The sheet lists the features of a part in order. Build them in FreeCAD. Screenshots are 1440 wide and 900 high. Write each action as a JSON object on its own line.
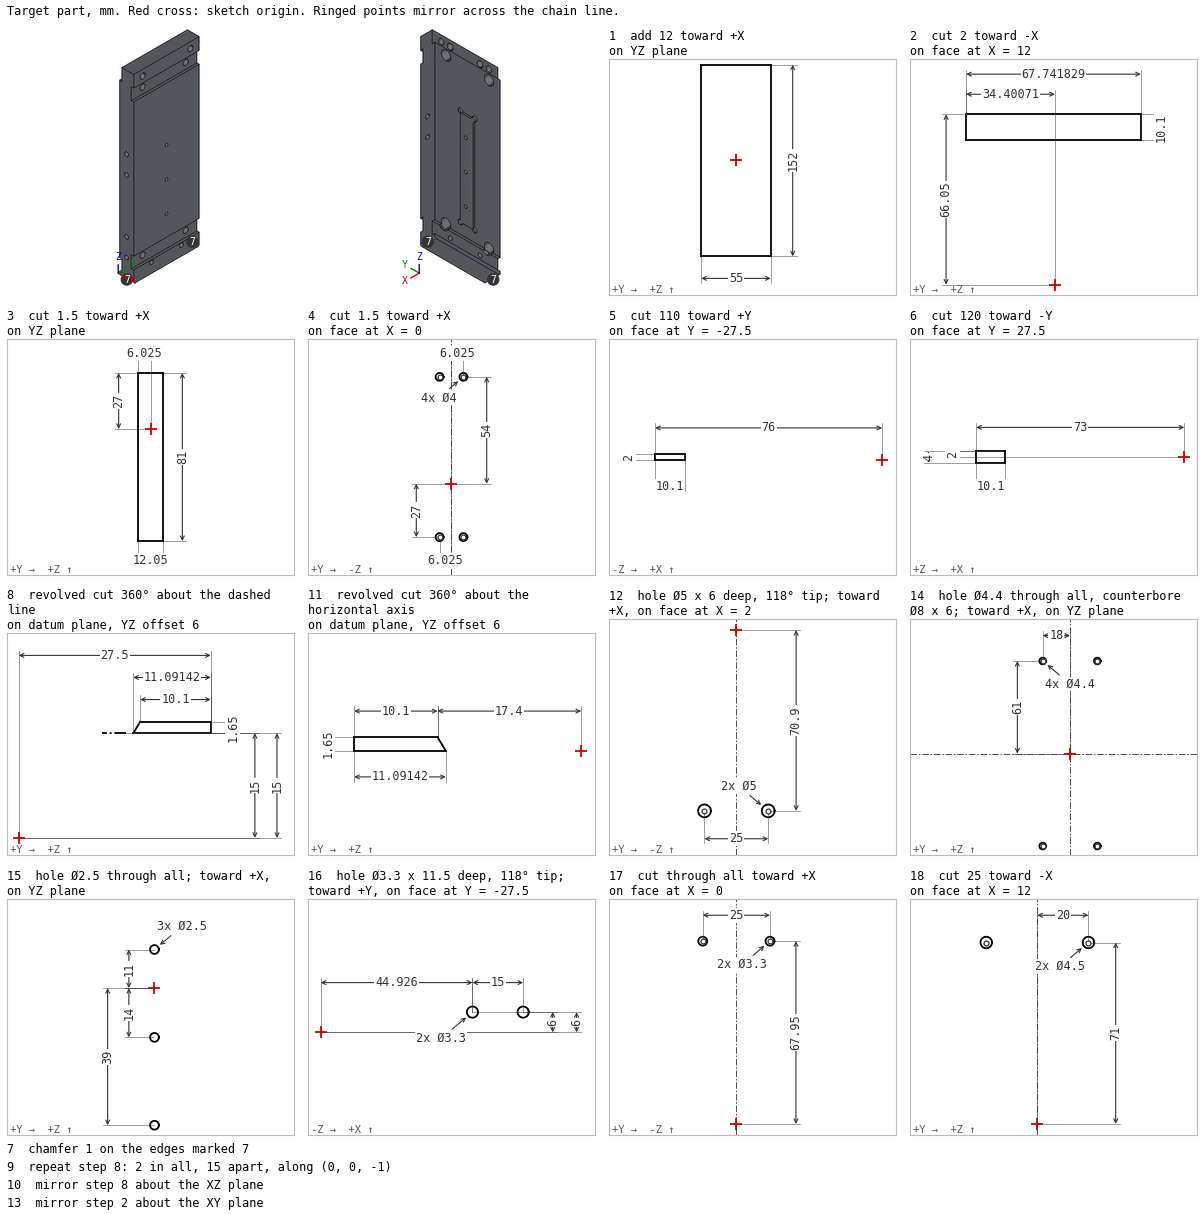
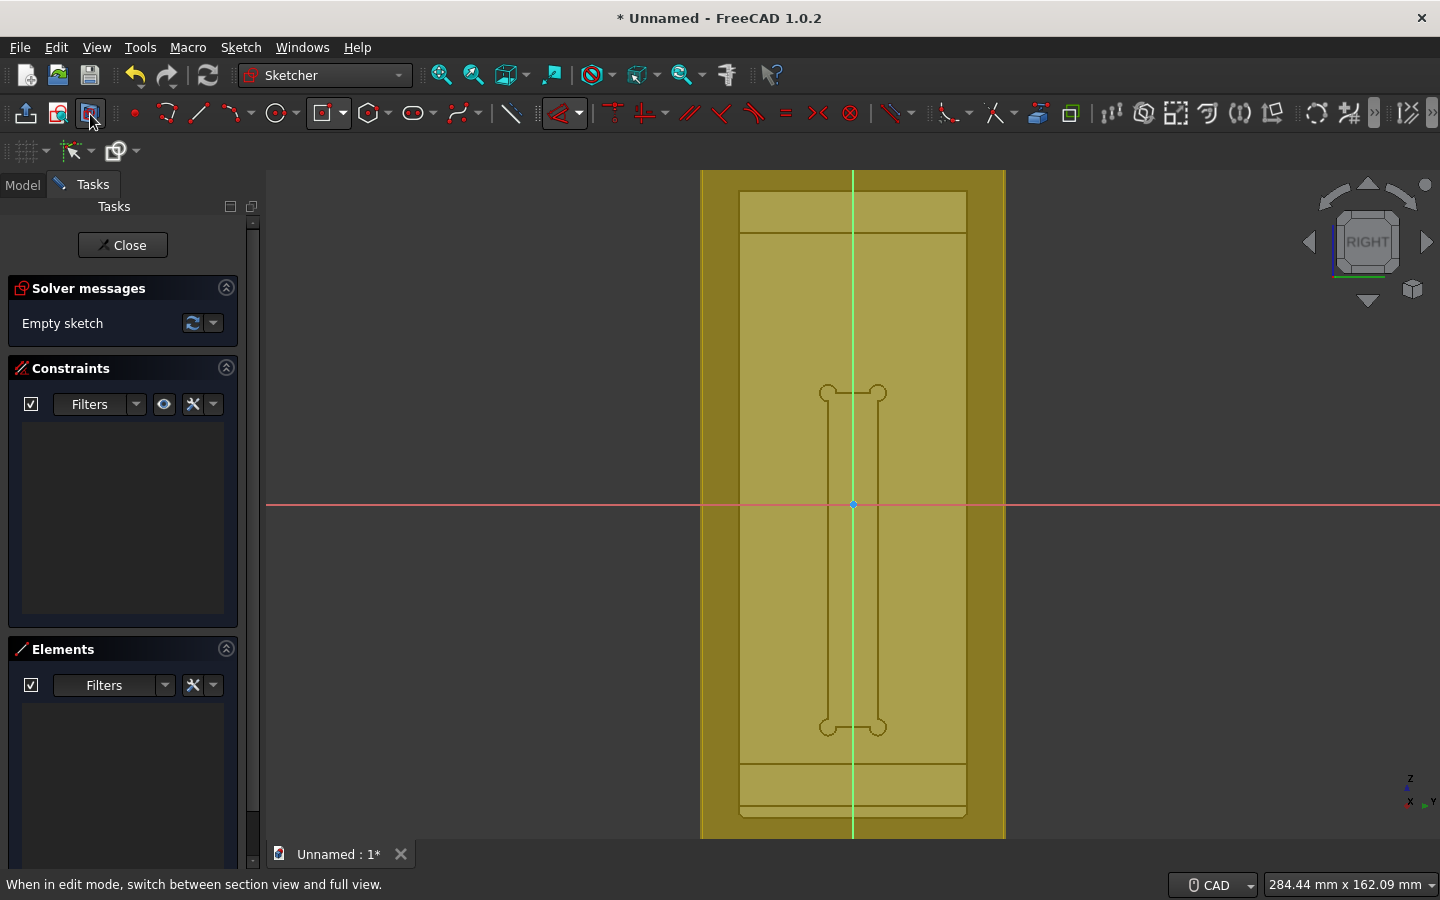
{"action": "scroll", "coordinate": [935, 463], "scroll_direction": "up", "scroll_amount": 9}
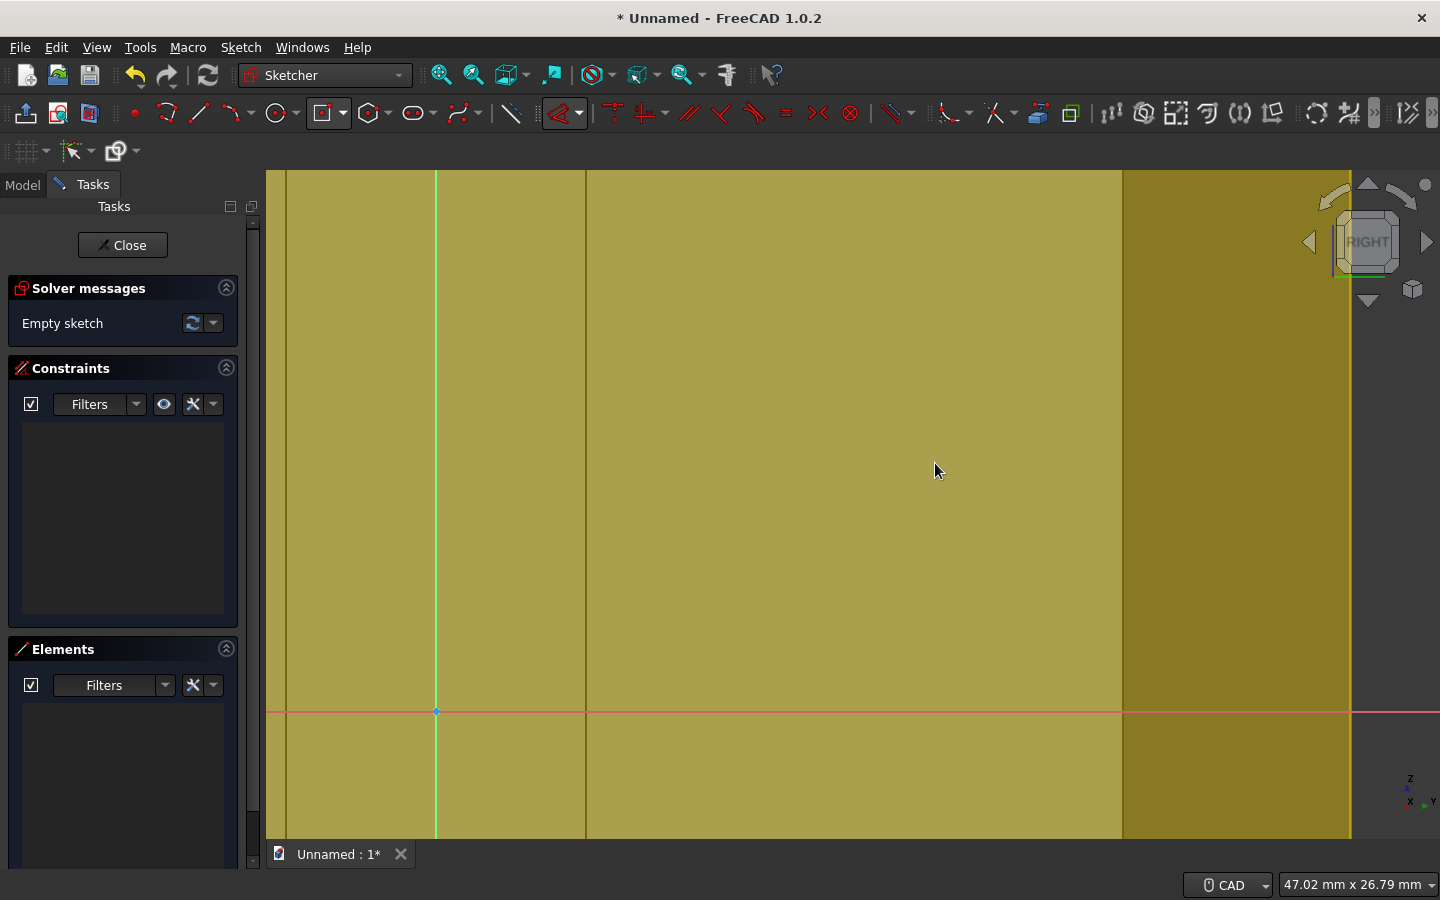
{"action": "left_click", "coordinate": [168, 114]}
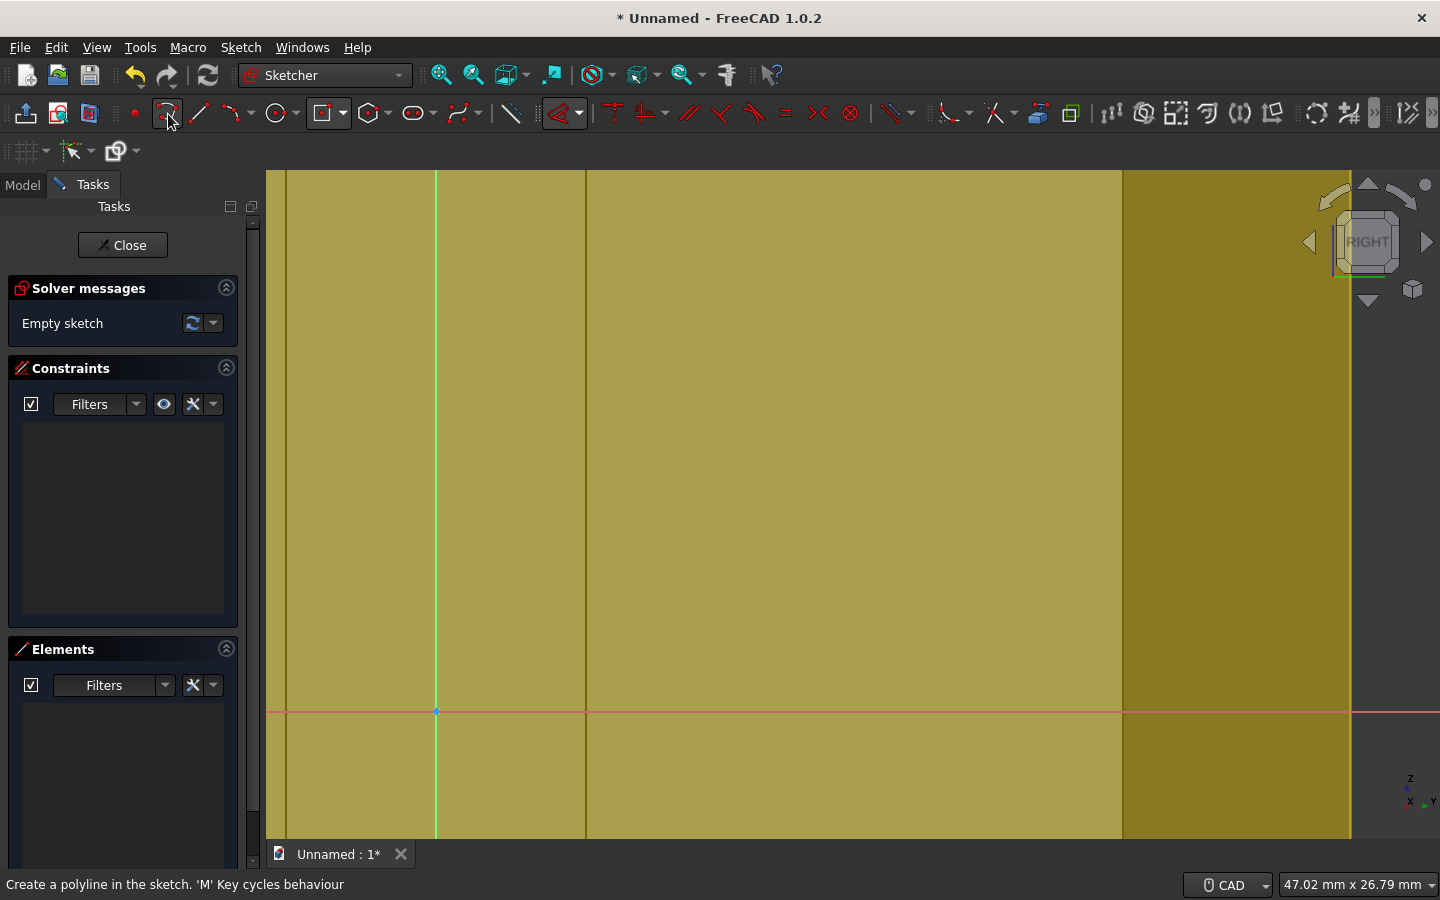
{"action": "left_click", "coordinate": [846, 337]}
{"action": "left_click", "coordinate": [1123, 337]}
{"action": "left_click", "coordinate": [1123, 296]}
{"action": "left_click", "coordinate": [871, 296]}
{"action": "left_click", "coordinate": [846, 338]}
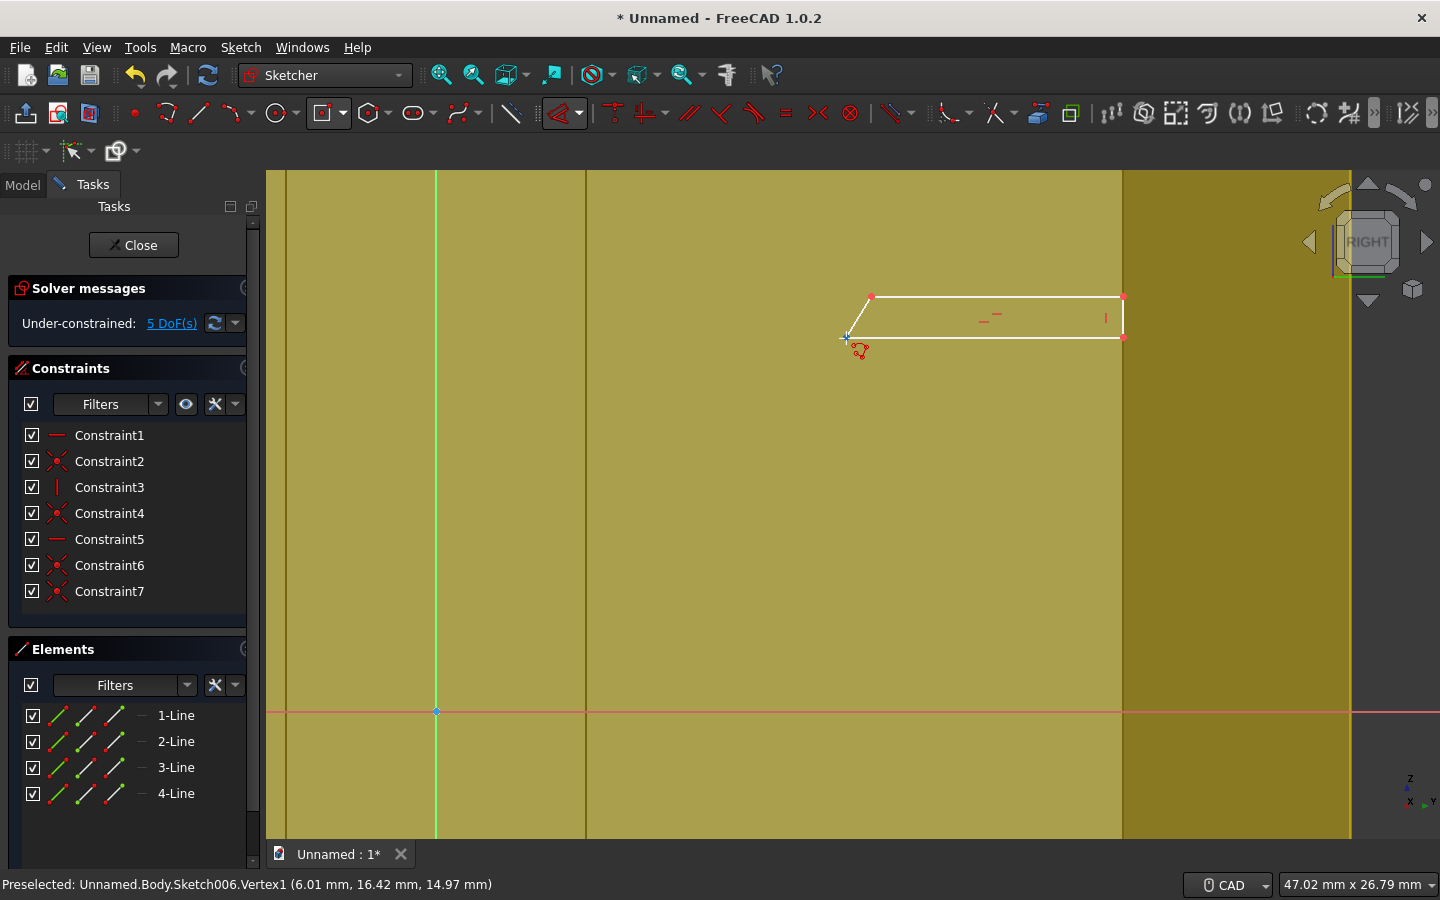
{"action": "left_click", "coordinate": [200, 114]}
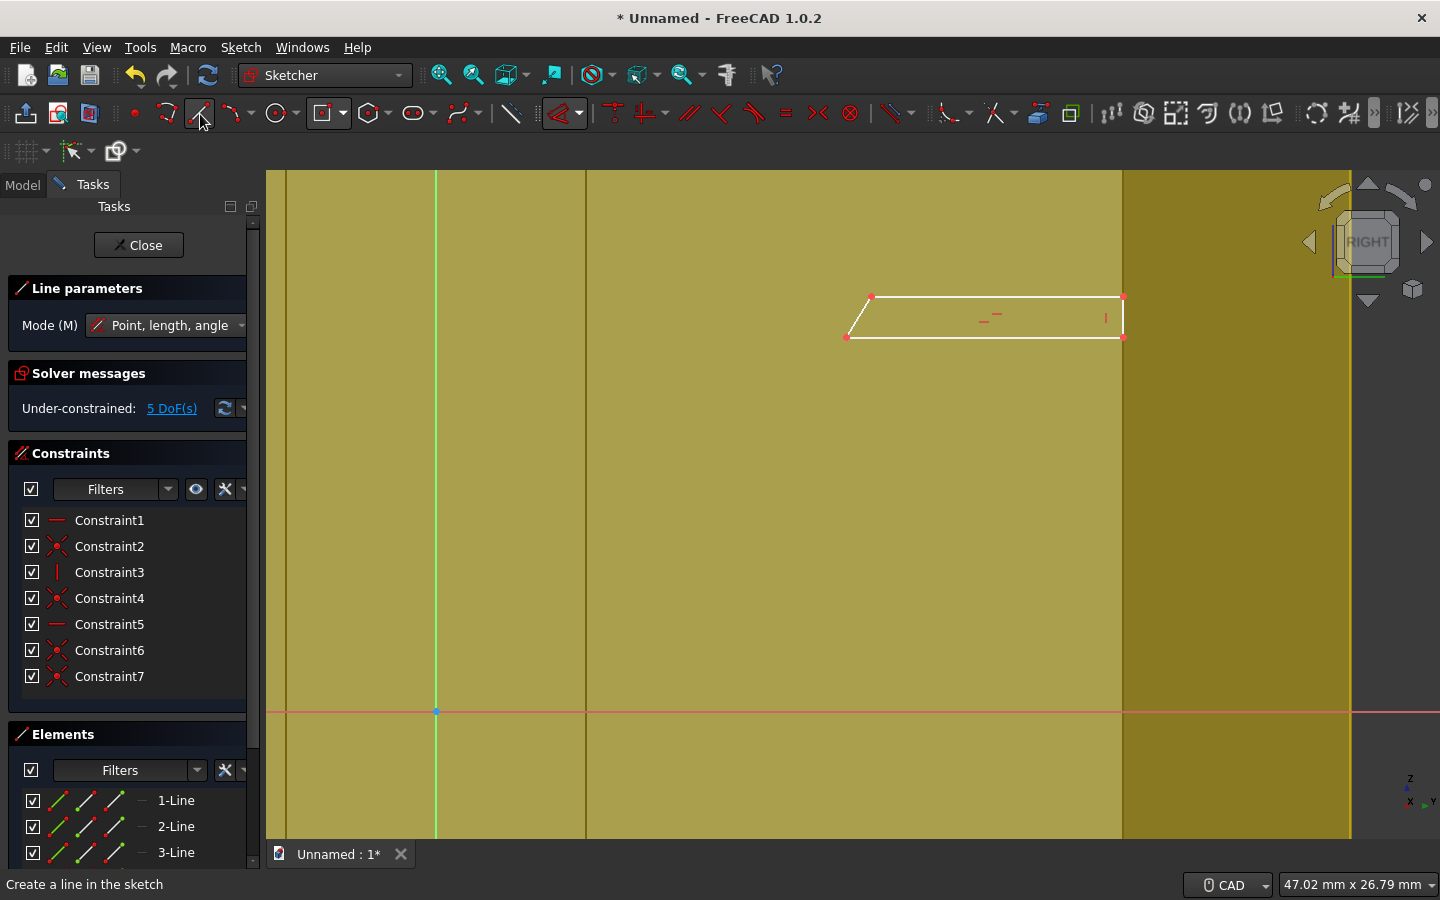
{"action": "left_click", "coordinate": [818, 337]}
{"action": "left_click", "coordinate": [735, 337]}
{"action": "key", "text": "Escape"}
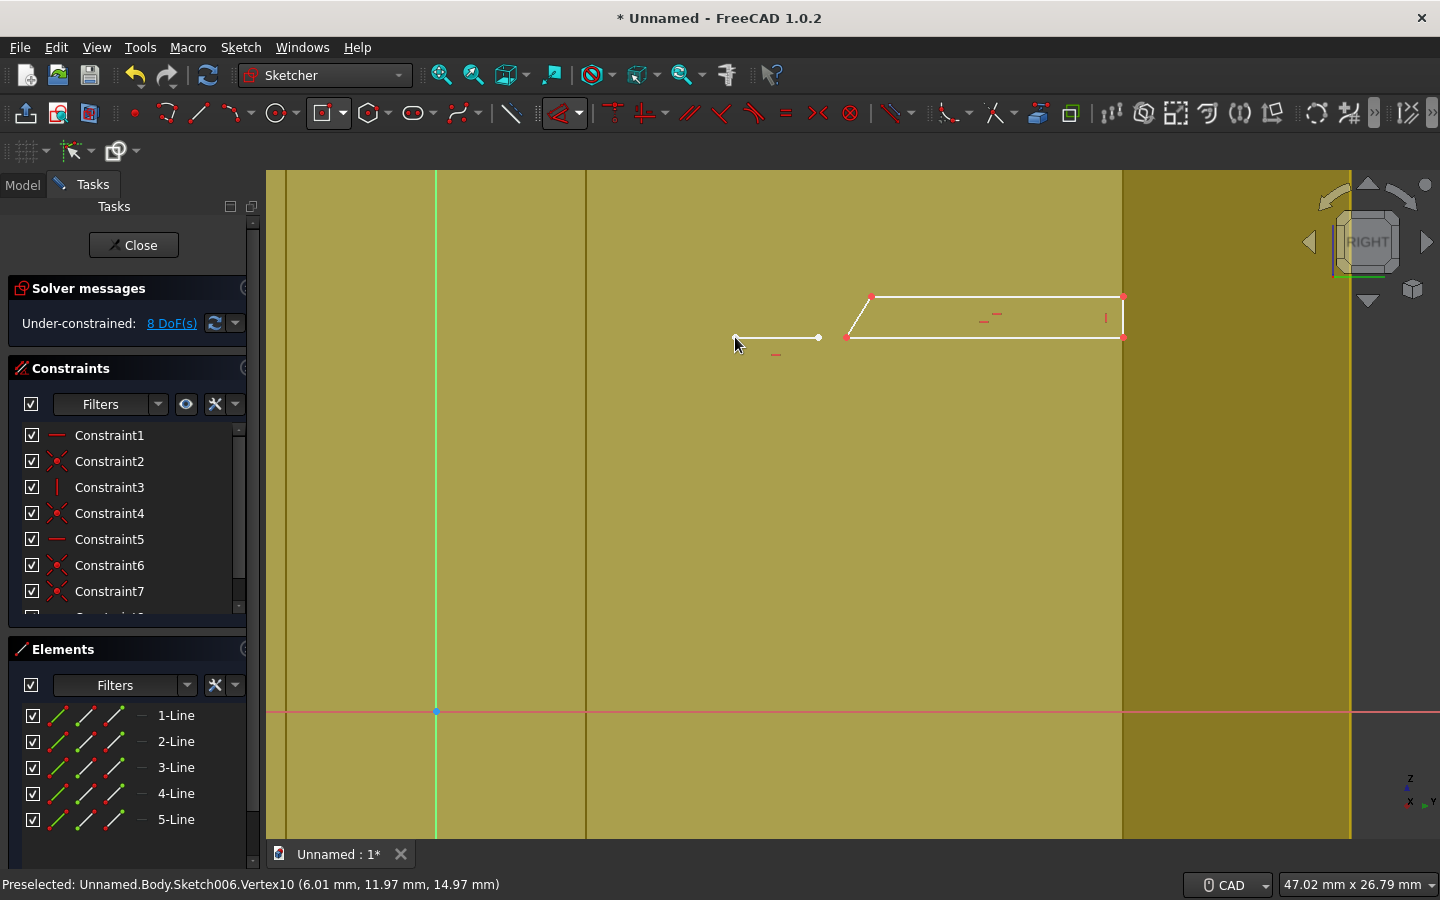
{"action": "left_click", "coordinate": [793, 338]}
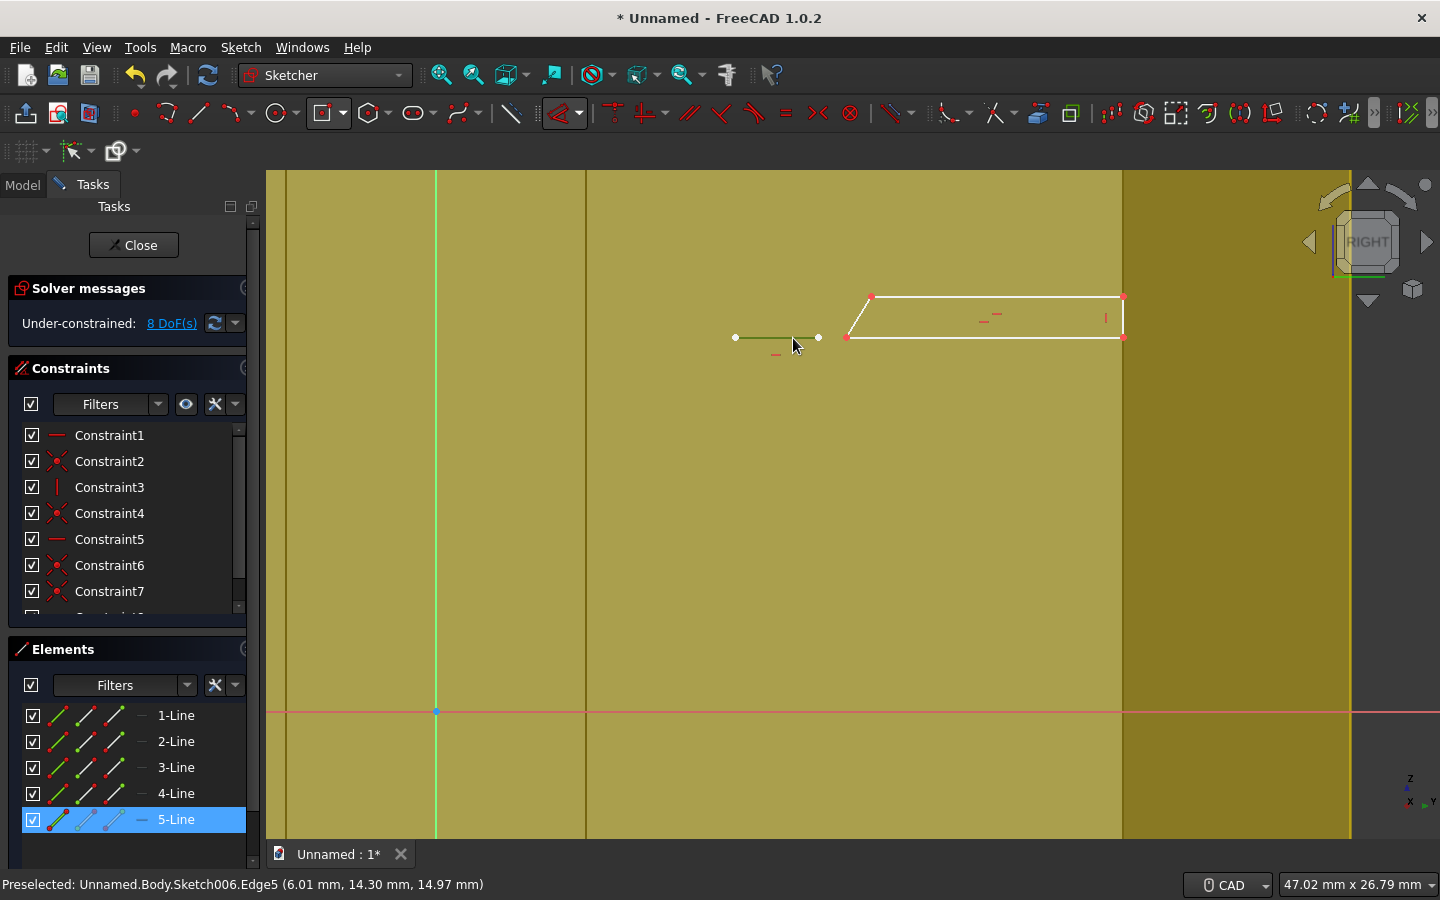
{"action": "left_click", "coordinate": [512, 114]}